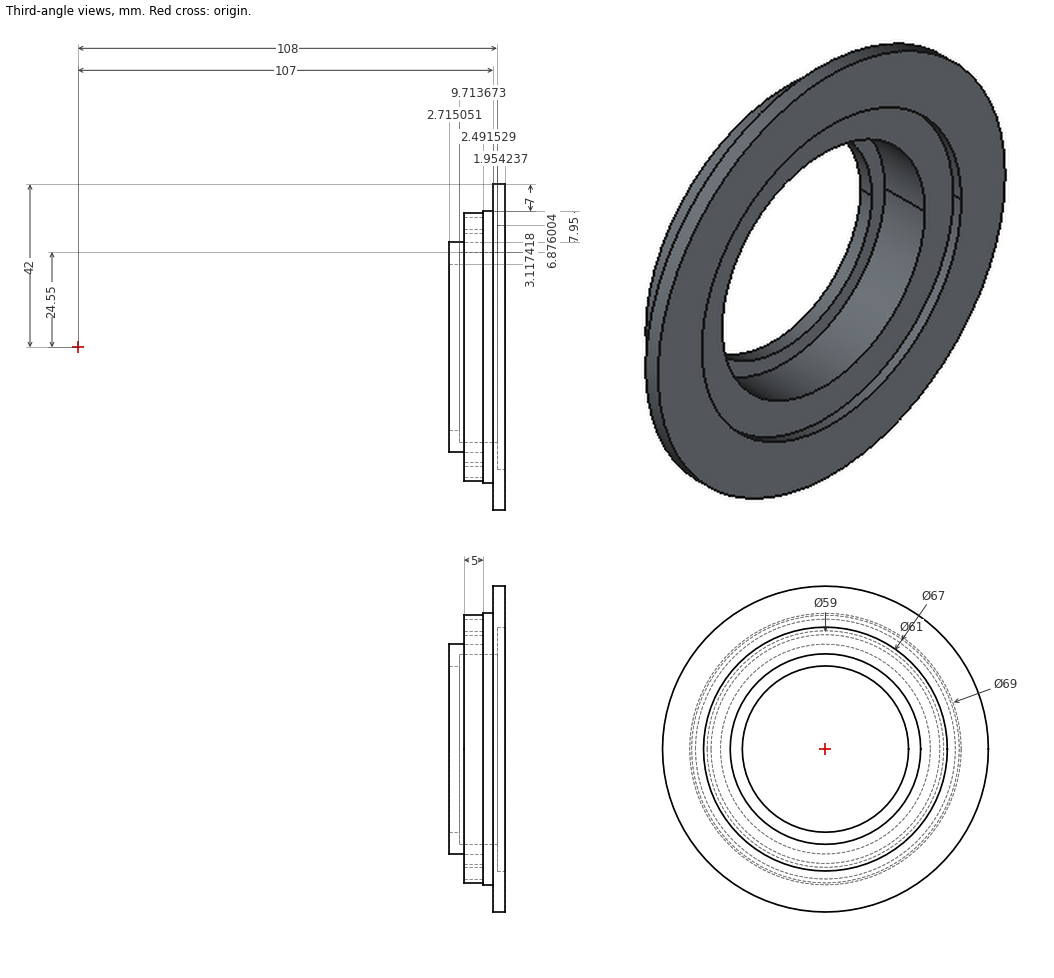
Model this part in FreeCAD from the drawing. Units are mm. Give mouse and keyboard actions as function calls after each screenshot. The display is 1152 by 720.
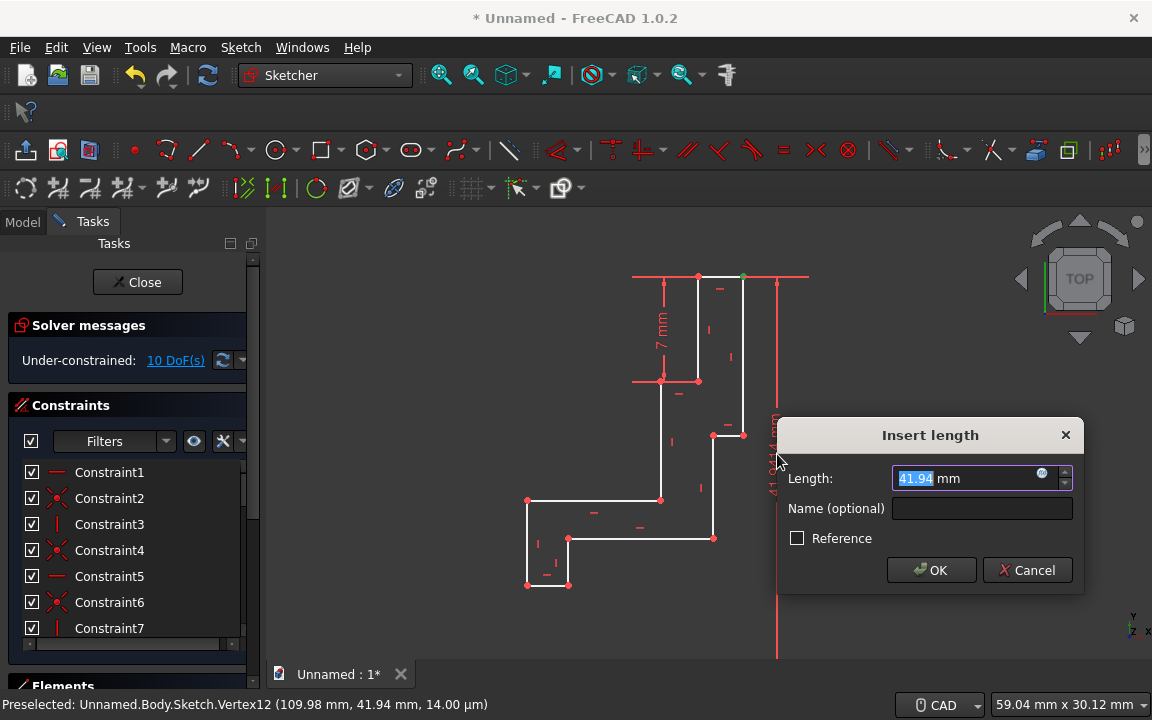
text(42)
key(Return)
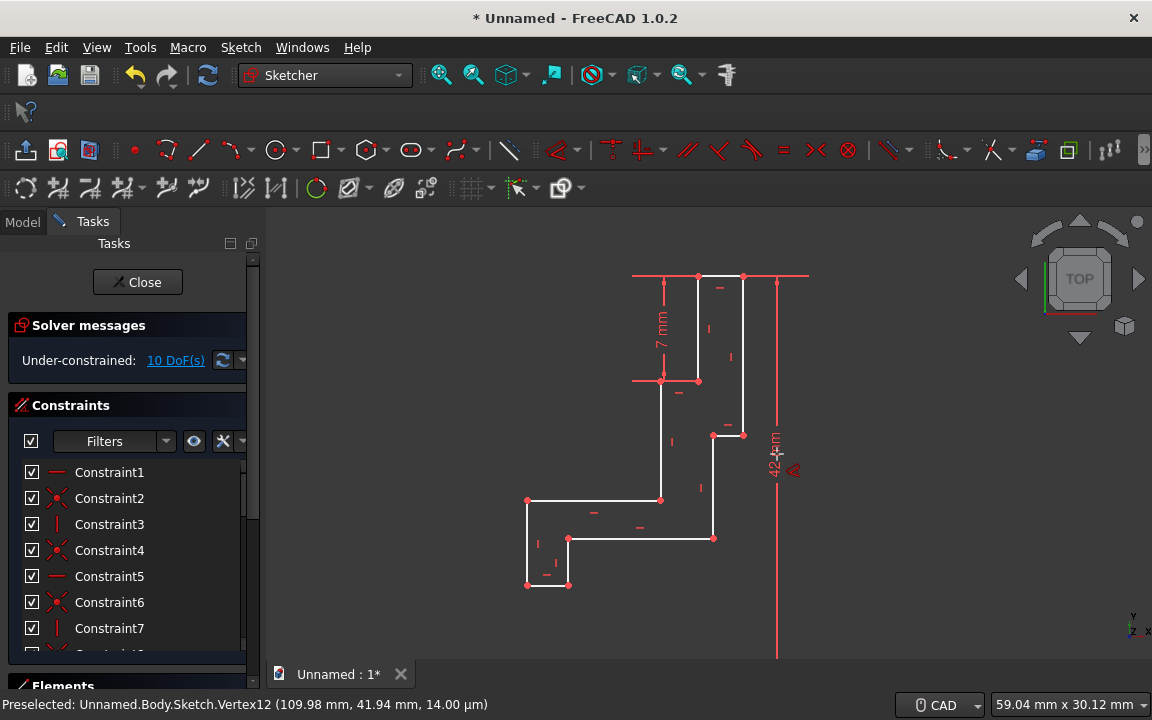
click(661, 417)
click(695, 441)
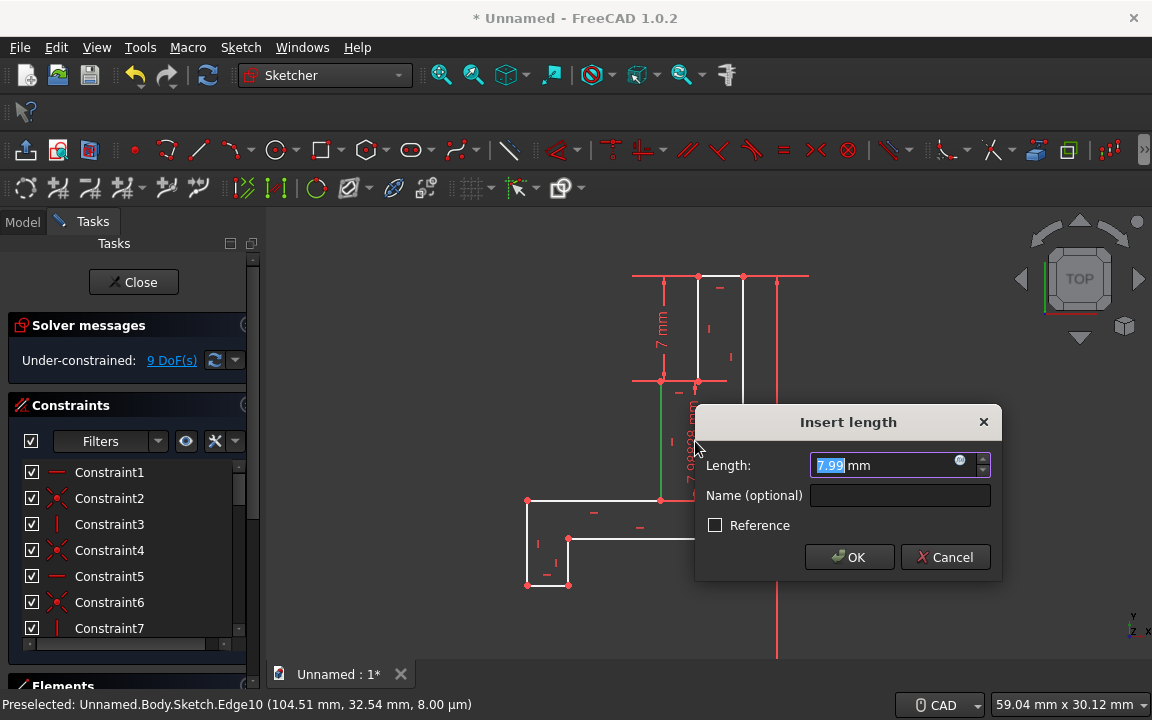
text(7.95)
key(Return)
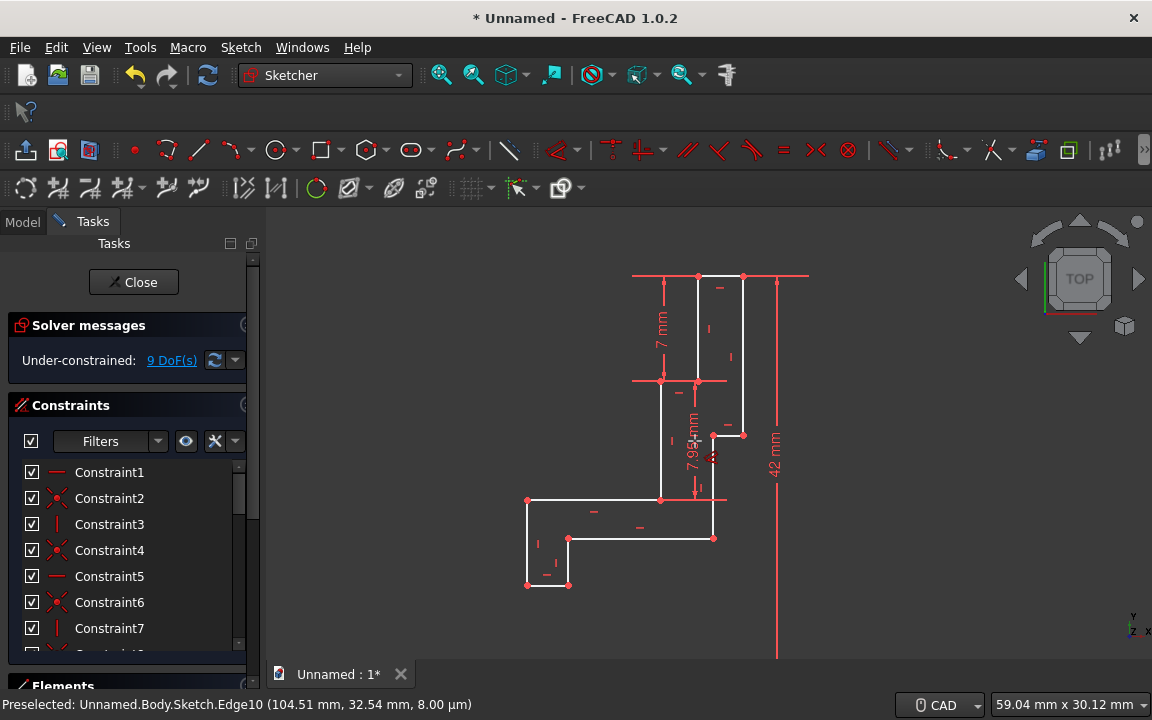
click(713, 539)
click(504, 505)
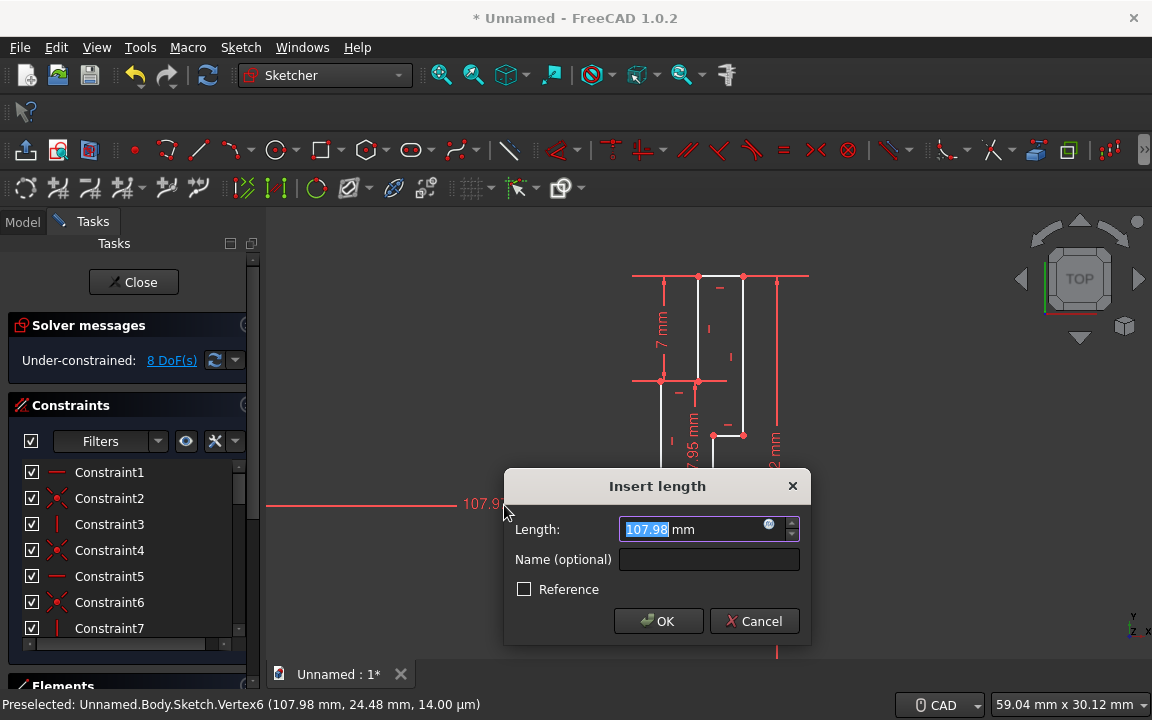
text(108)
key(Return)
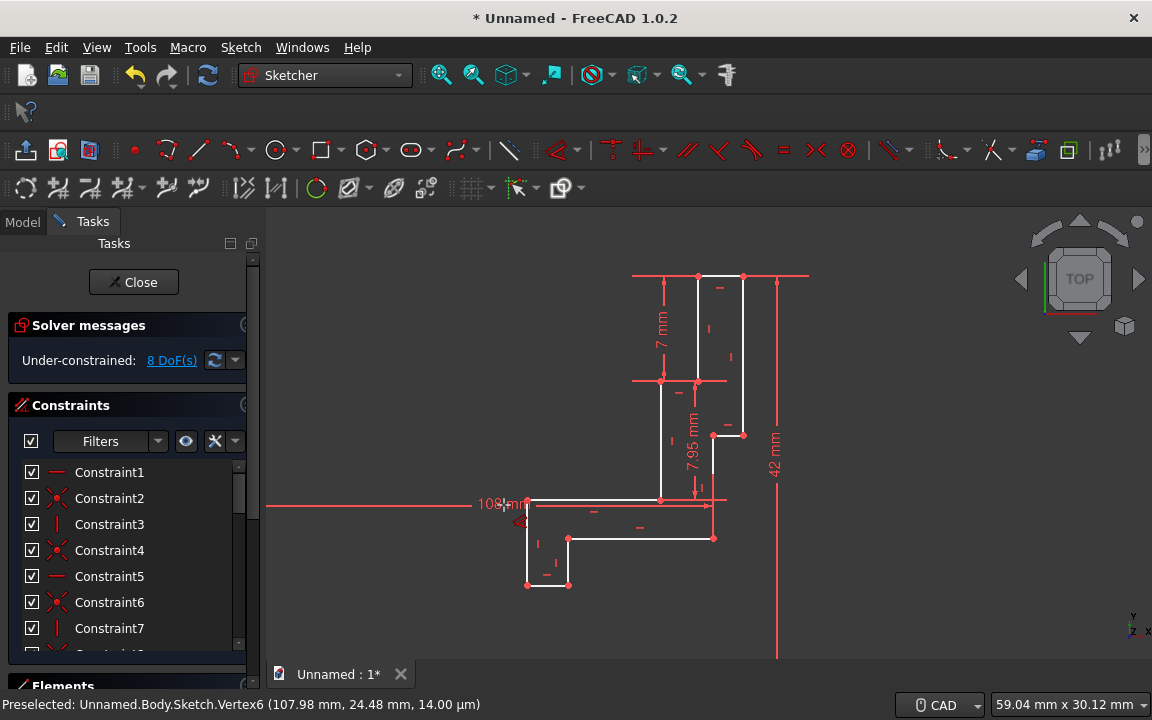
click(698, 276)
click(496, 242)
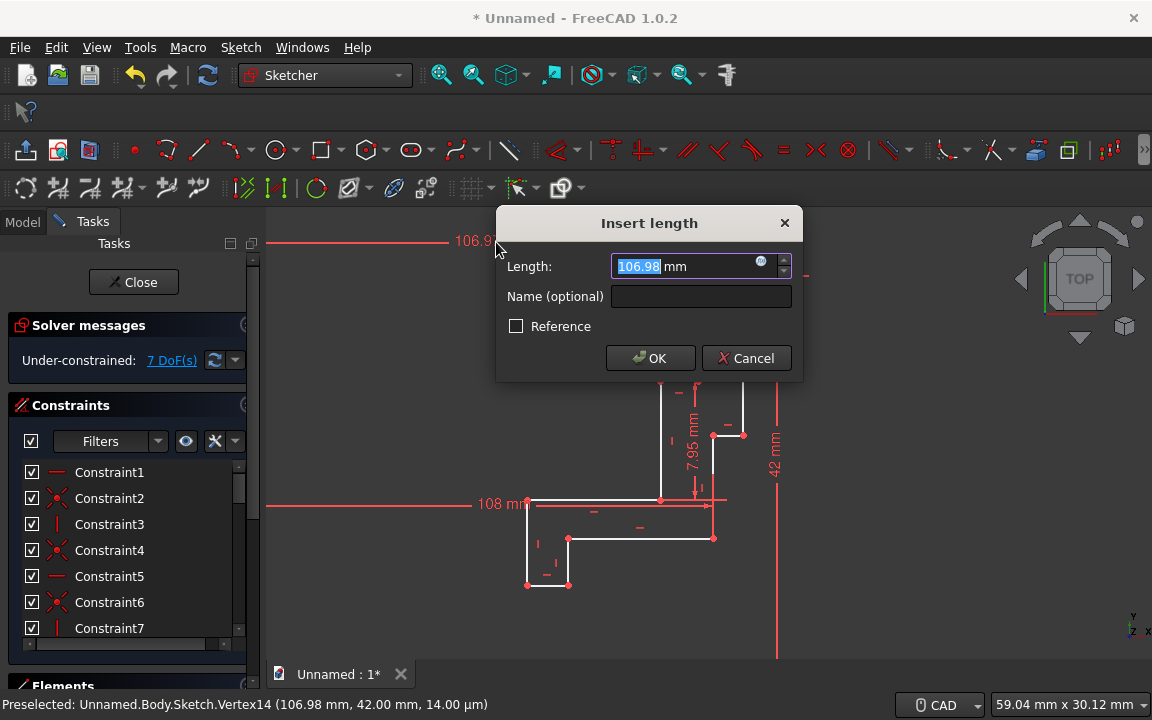
text(107)
key(Return)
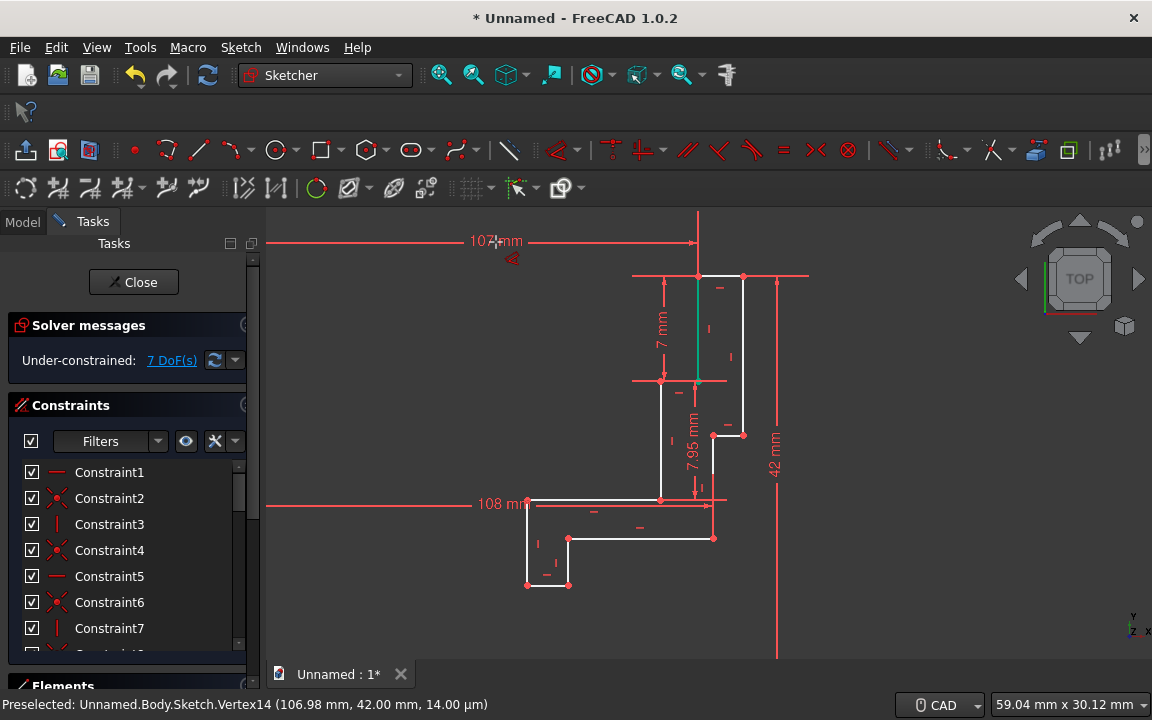
click(568, 539)
click(602, 585)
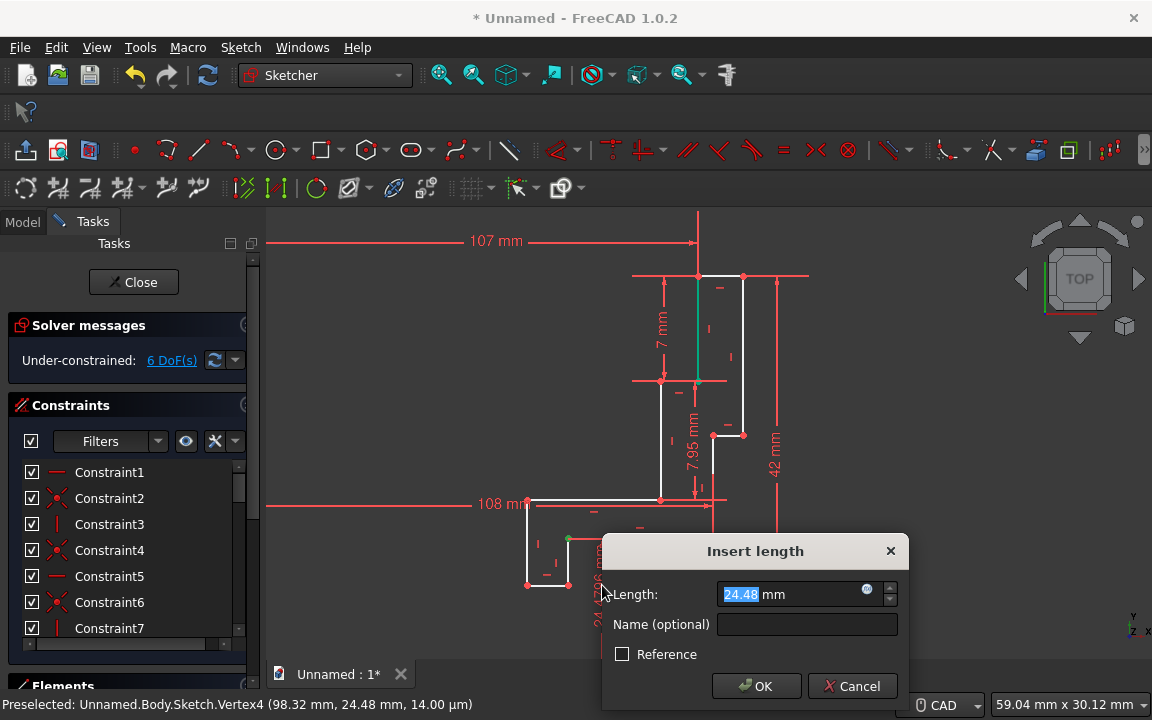
text(24.55)
key(Return)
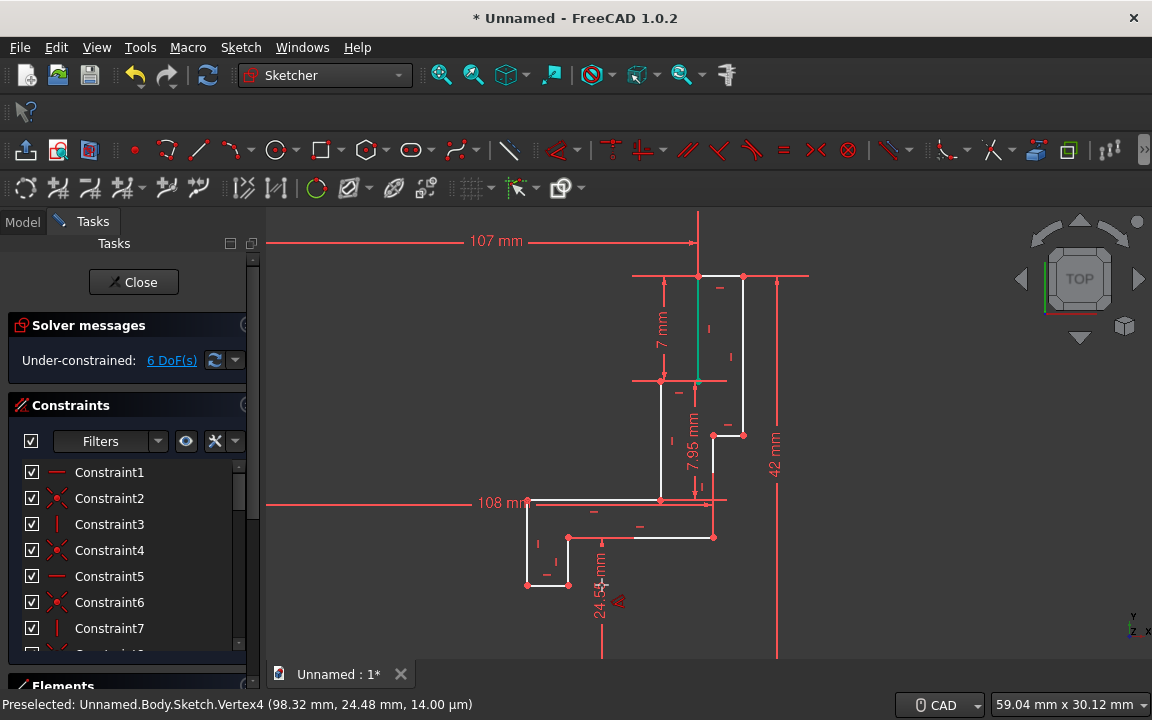
click(539, 586)
click(548, 620)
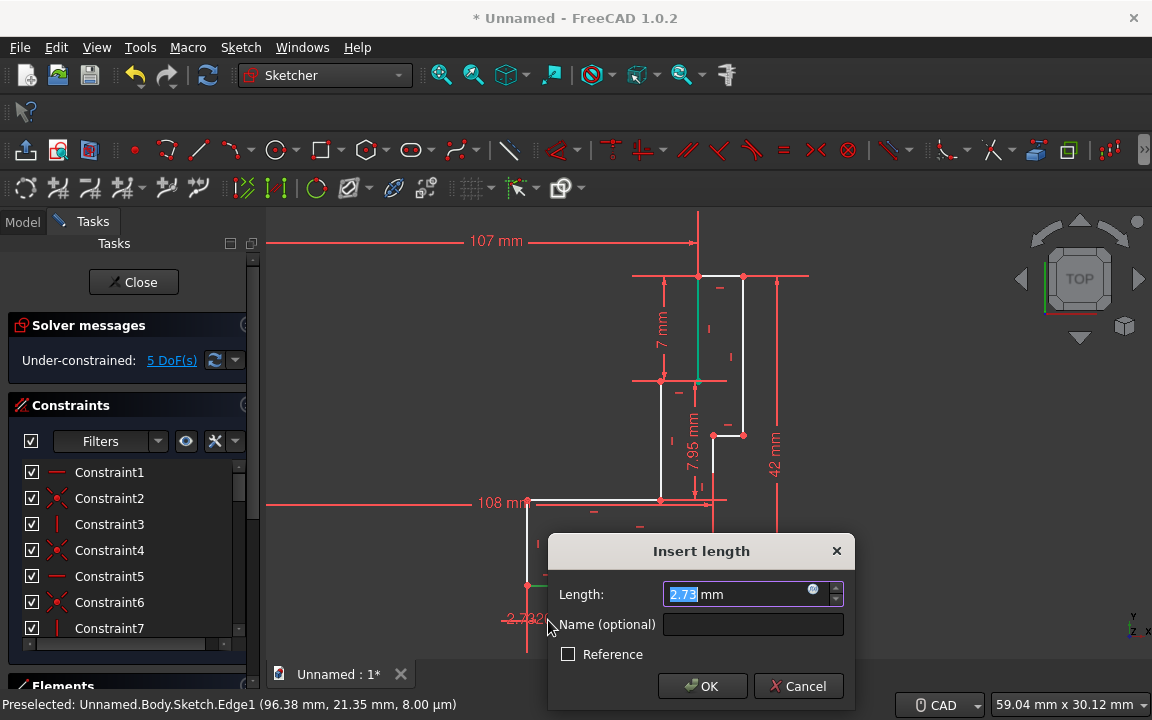
text(2.715051)
key(Return)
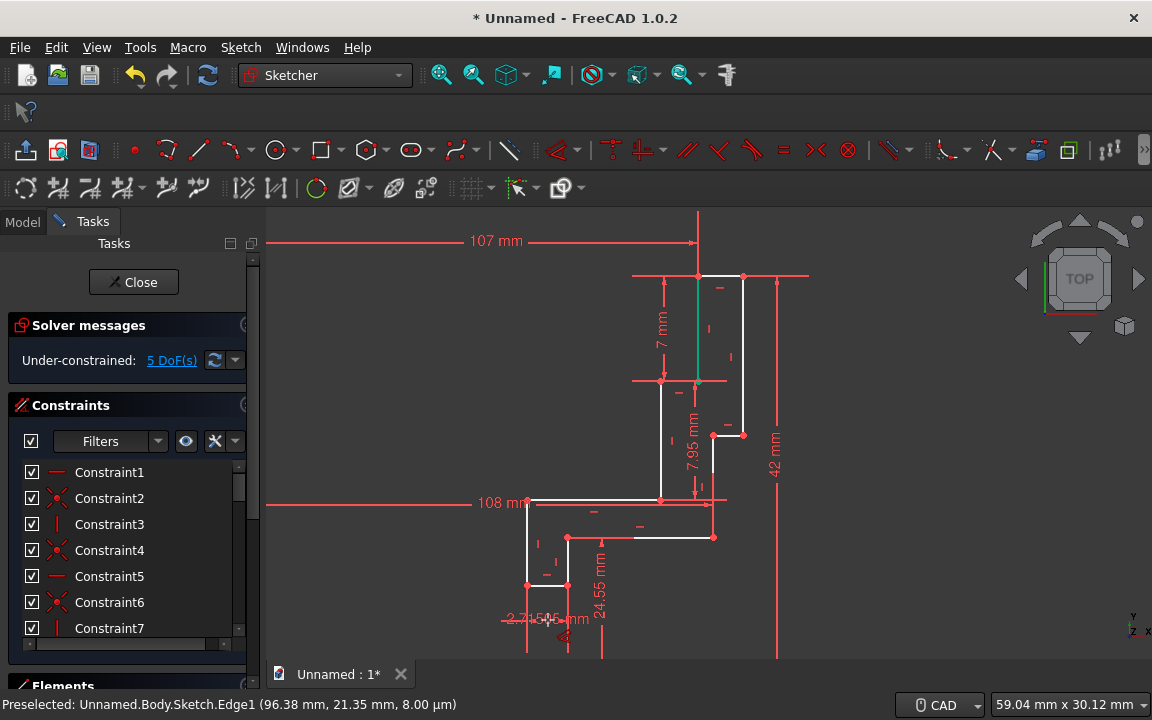
click(568, 572)
click(602, 562)